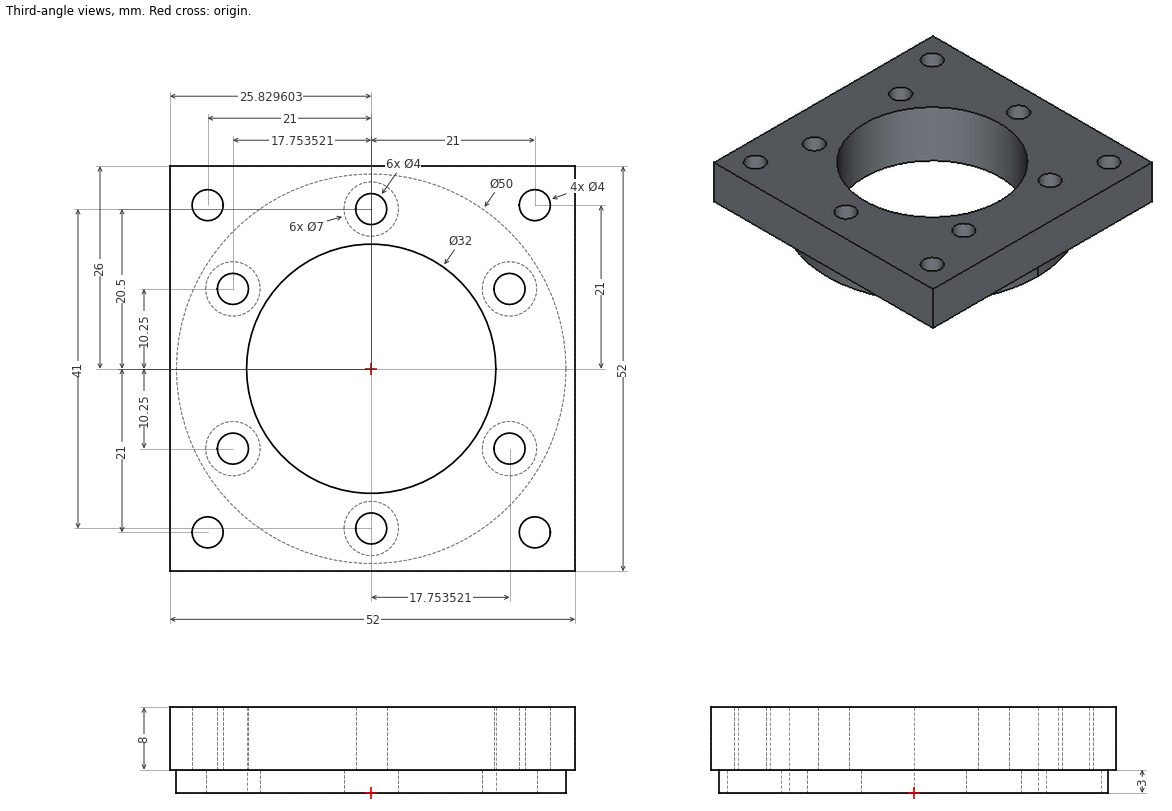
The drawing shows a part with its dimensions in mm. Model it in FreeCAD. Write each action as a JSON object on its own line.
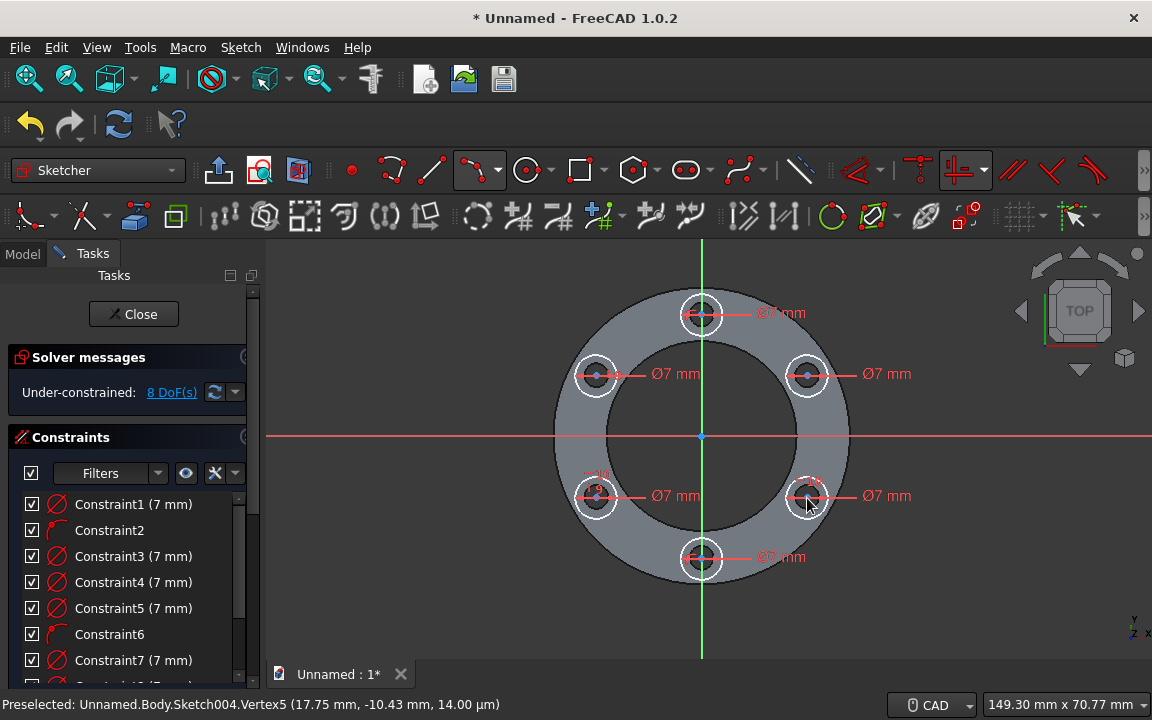
{"action": "left_click", "coordinate": [807, 498]}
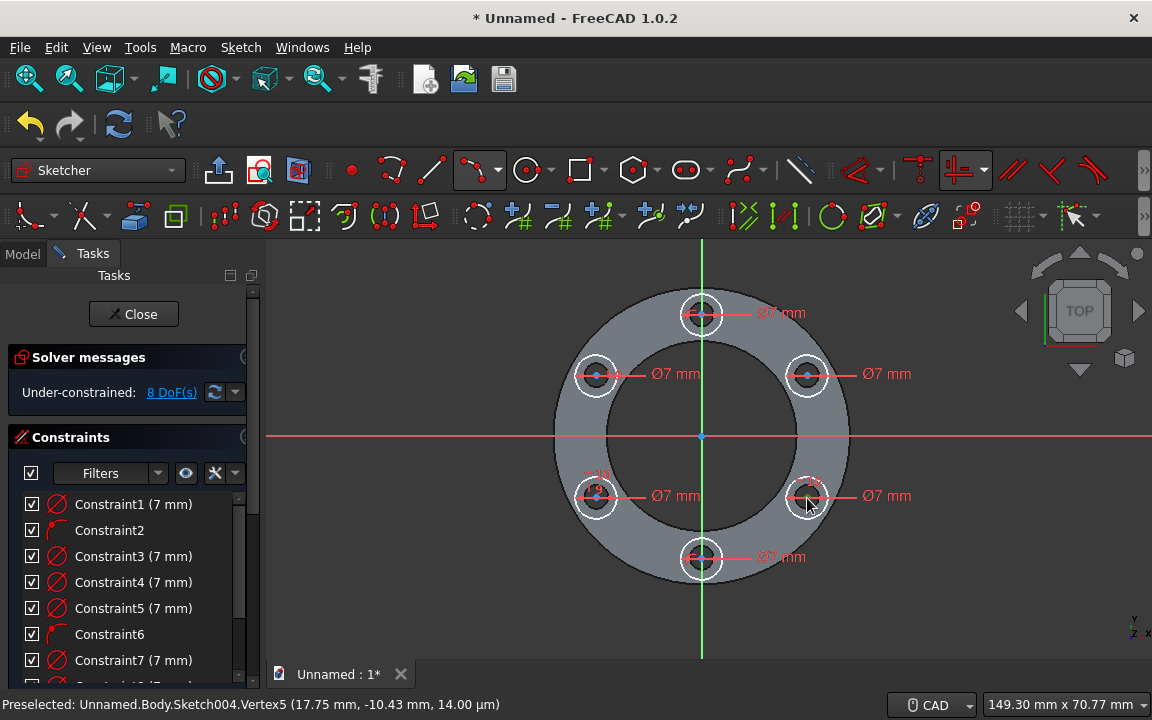
{"action": "left_click", "coordinate": [807, 376]}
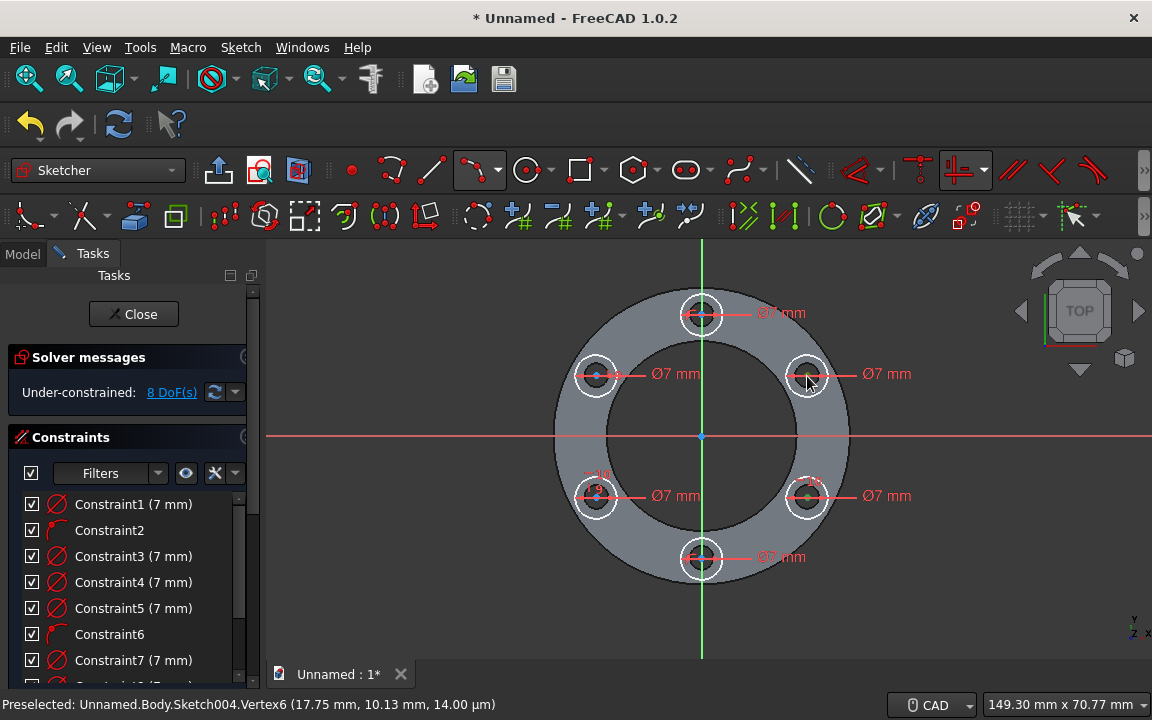
{"action": "key", "text": "v"}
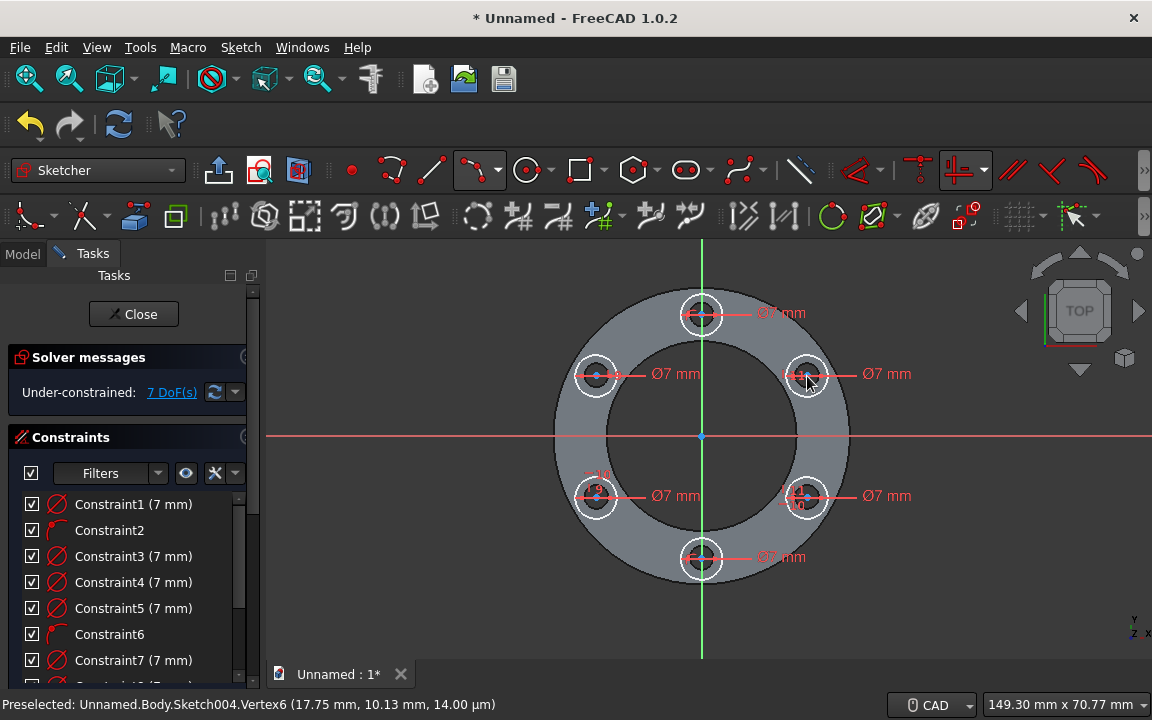
{"action": "left_click", "coordinate": [596, 376]}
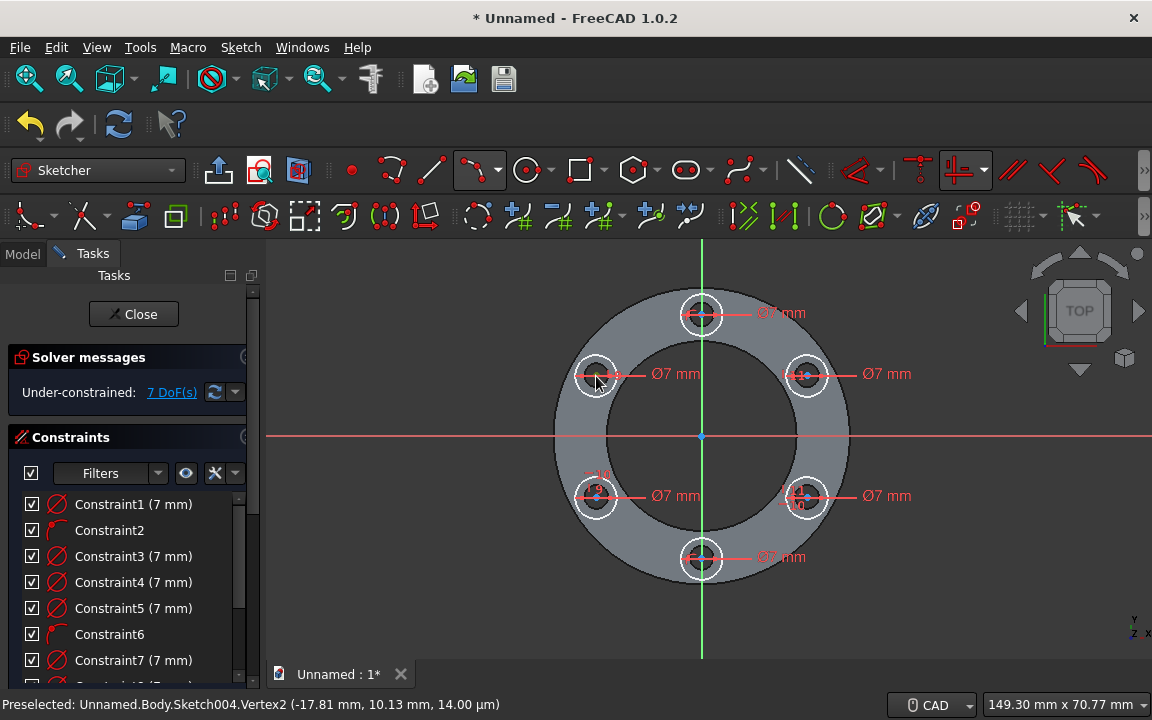
{"action": "left_click", "coordinate": [807, 376]}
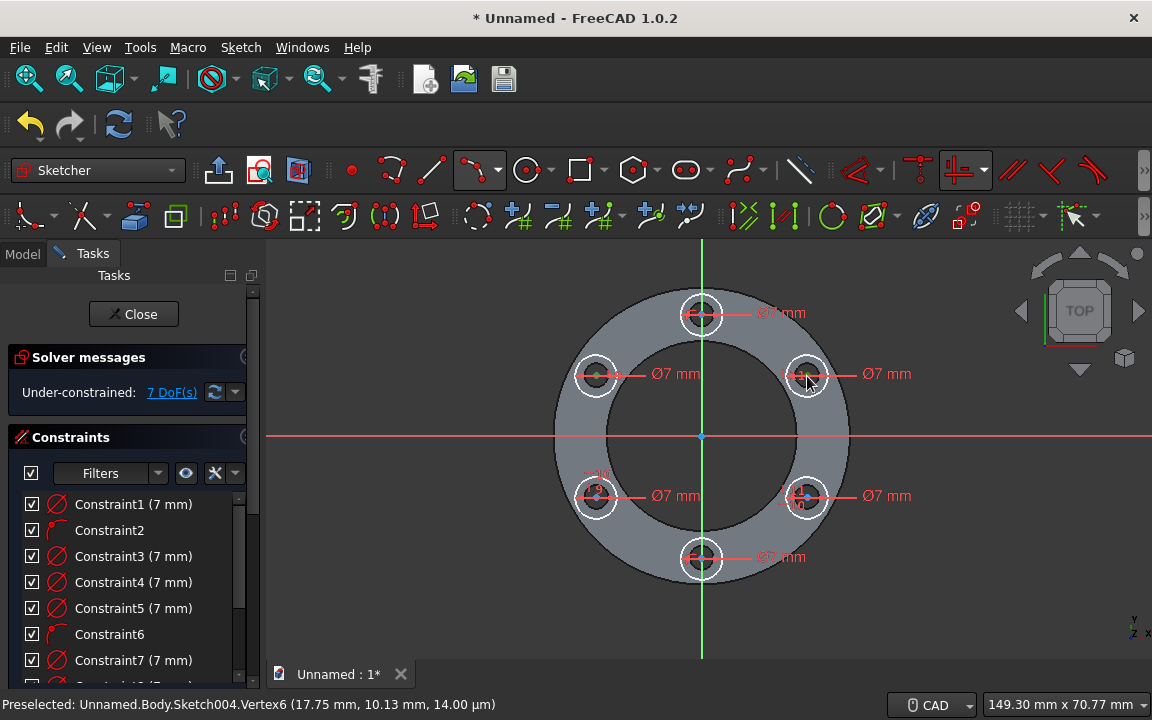
{"action": "key", "text": "h"}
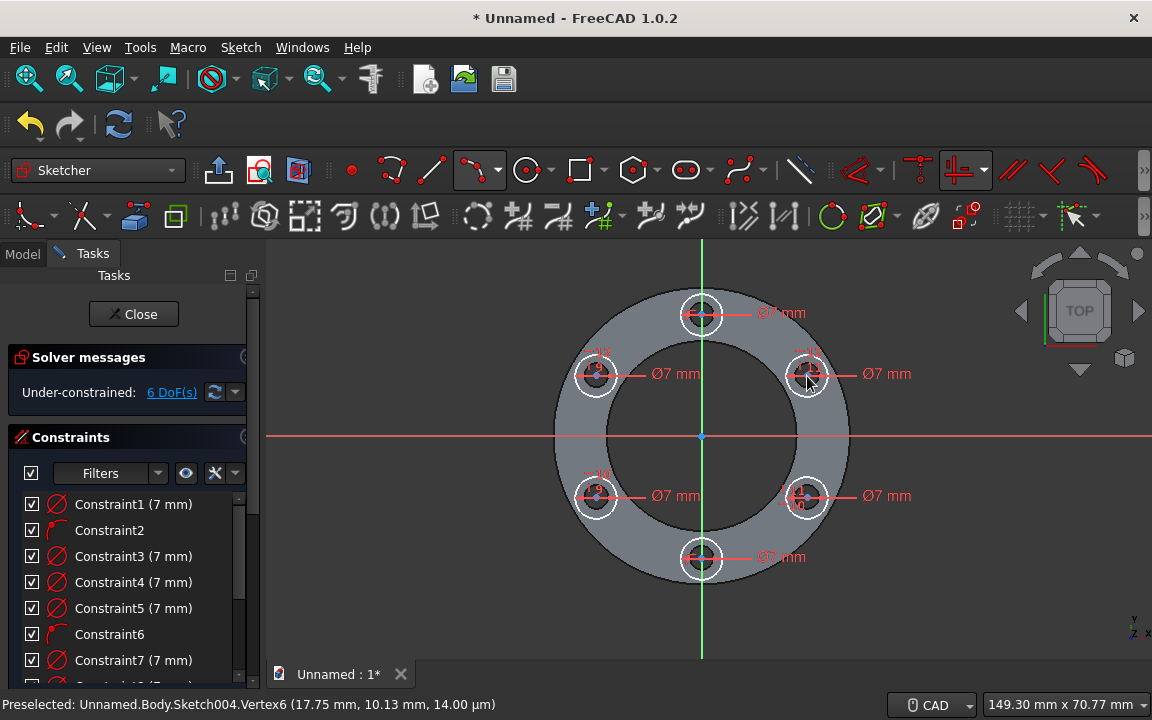
{"action": "key", "text": "d"}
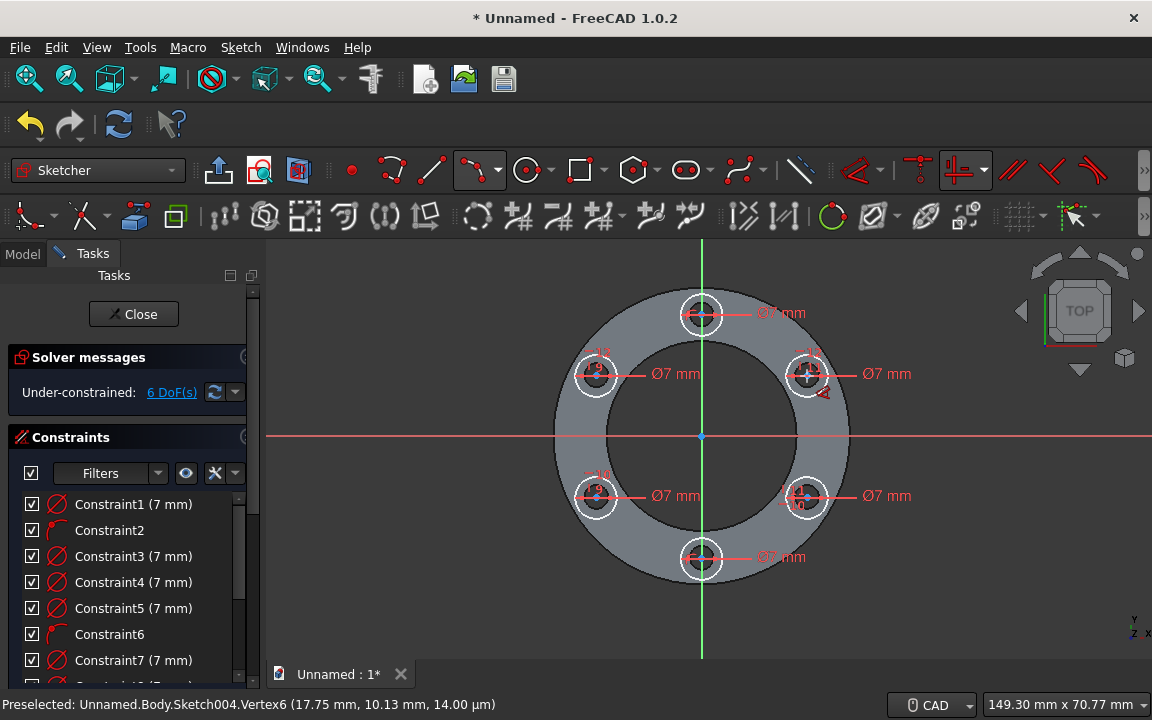
{"action": "left_click", "coordinate": [702, 315]}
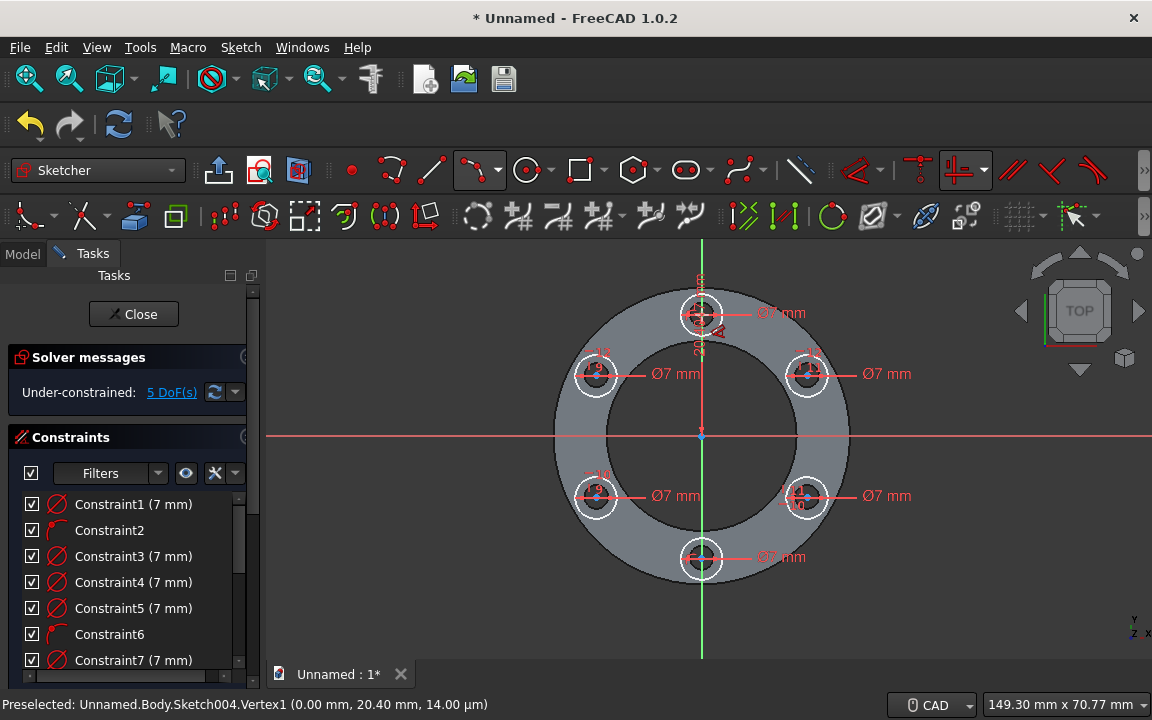
{"action": "left_click", "coordinate": [702, 559]}
{"action": "left_click", "coordinate": [736, 381]}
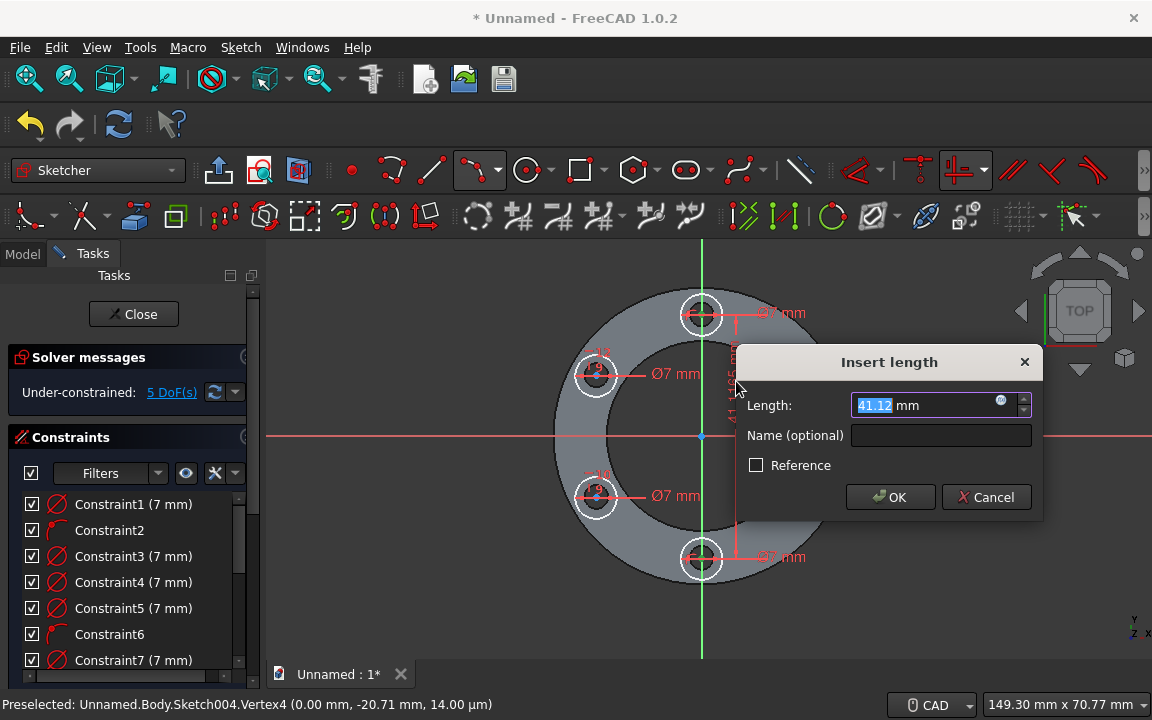
{"action": "type", "text": "41"}
{"action": "key", "text": "Return"}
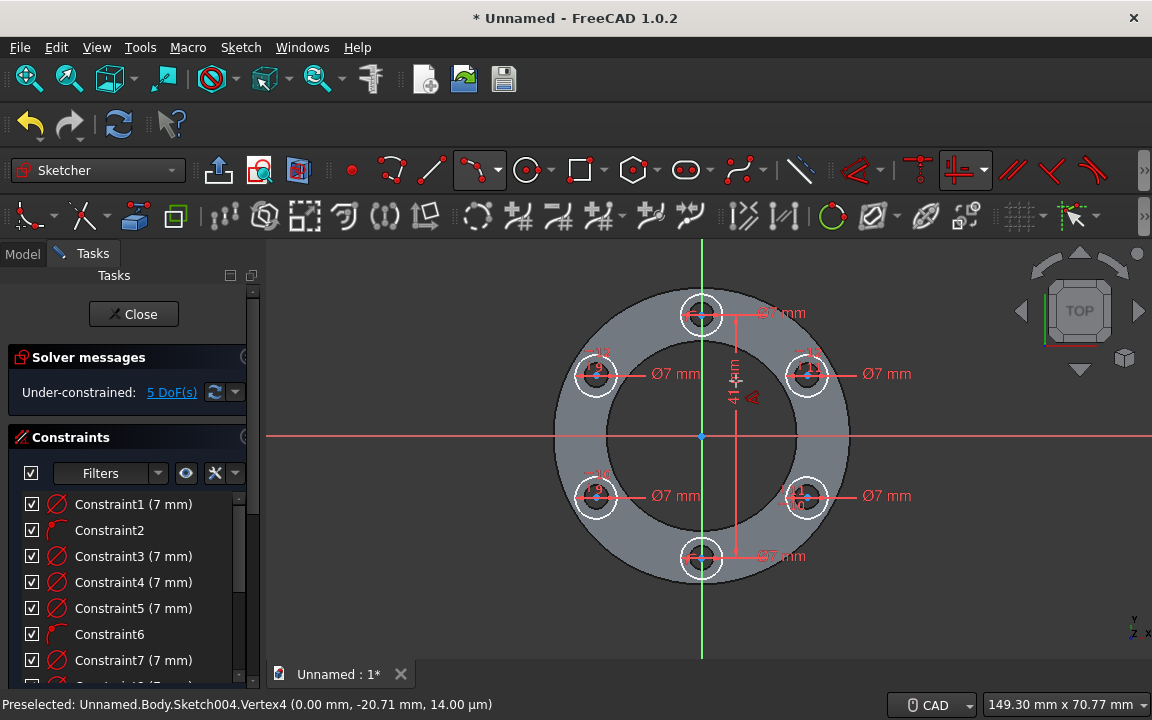
{"action": "left_click", "coordinate": [702, 315]}
{"action": "left_click", "coordinate": [736, 348]}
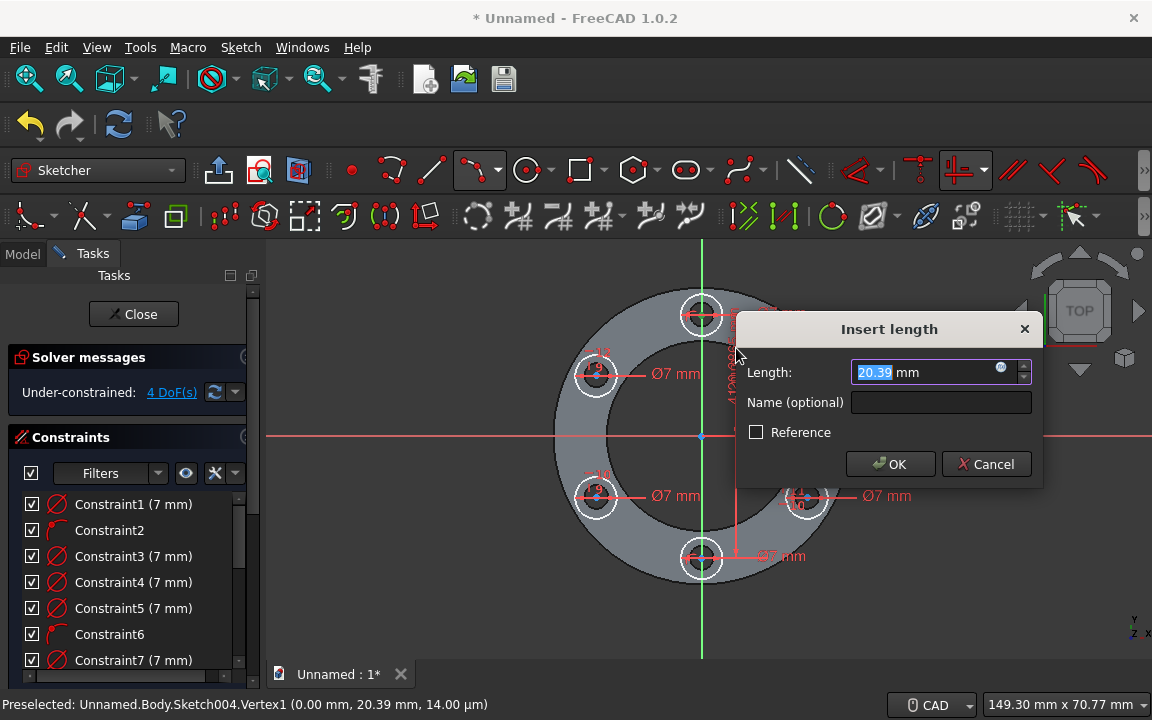
{"action": "type", "text": "20.5"}
{"action": "key", "text": "Return"}